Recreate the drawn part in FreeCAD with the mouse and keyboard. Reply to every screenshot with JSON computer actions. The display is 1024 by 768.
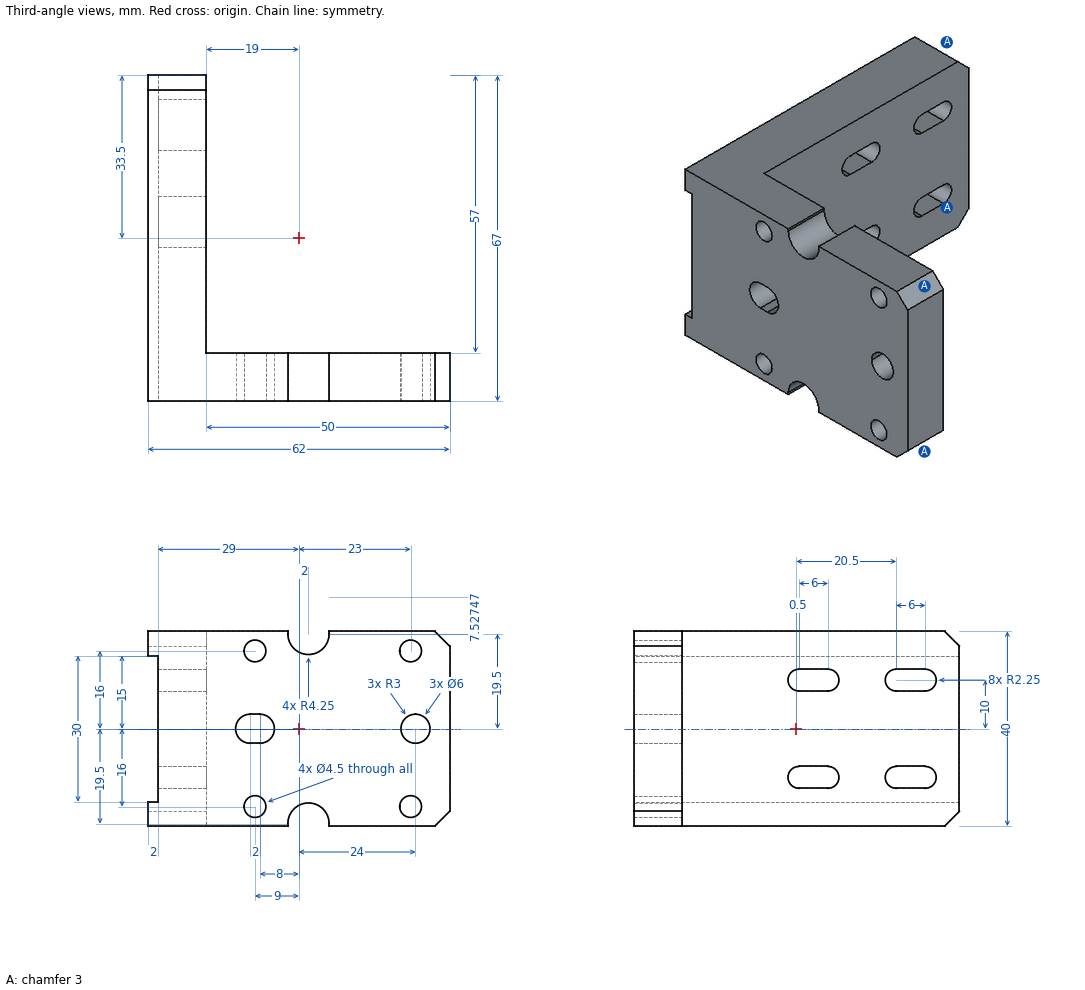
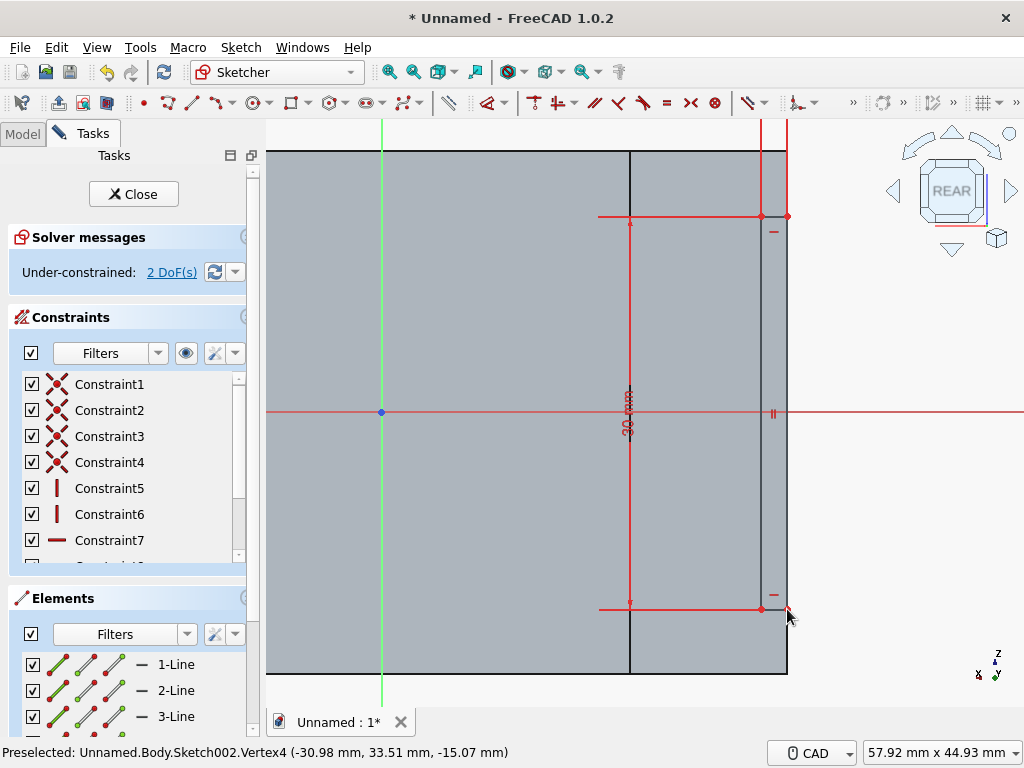
{"action": "left_click", "coordinate": [488, 104]}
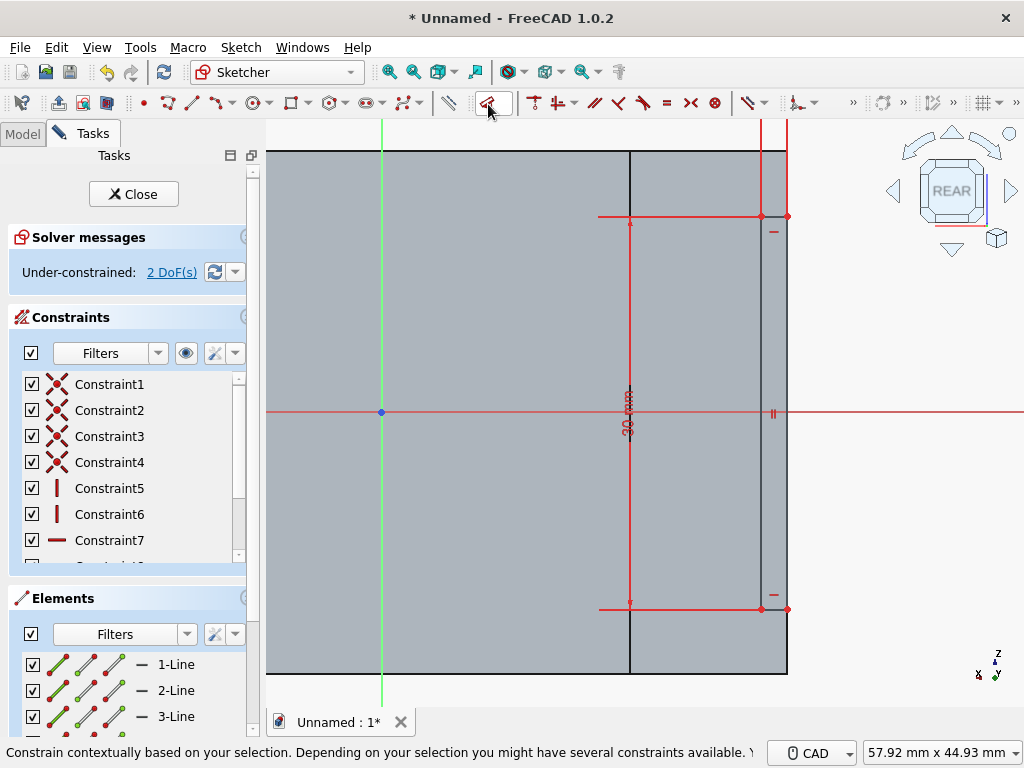
{"action": "left_click", "coordinate": [761, 217]}
{"action": "left_click", "coordinate": [571, 183]}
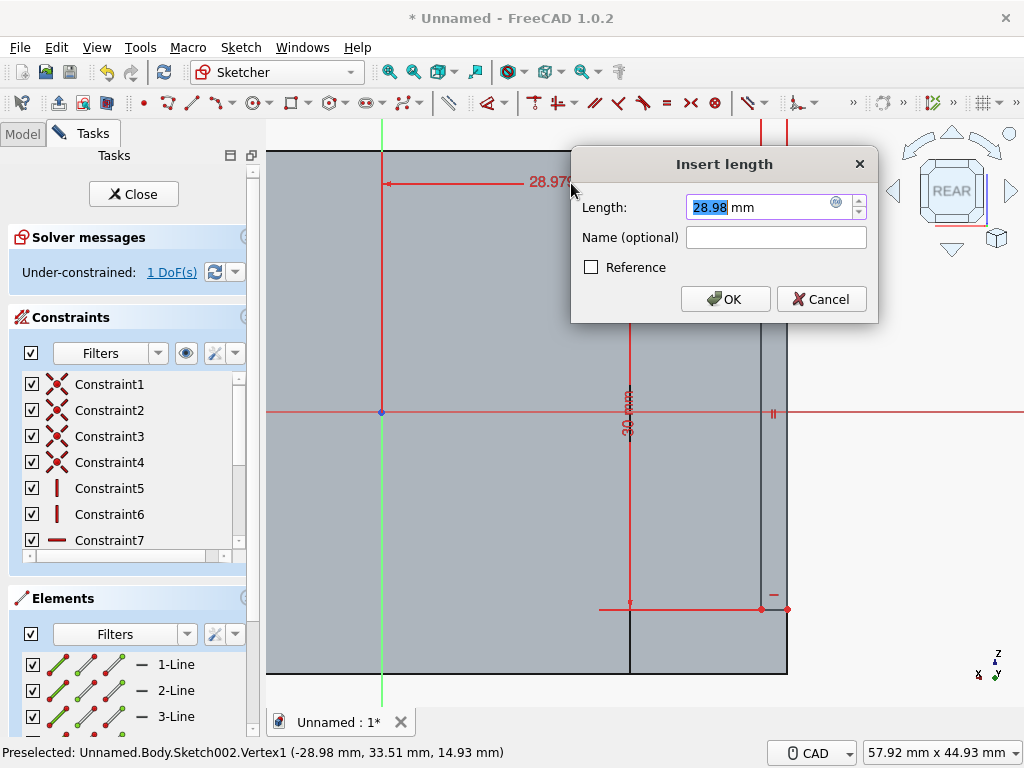
{"action": "type", "text": "29"}
{"action": "key", "text": "Return"}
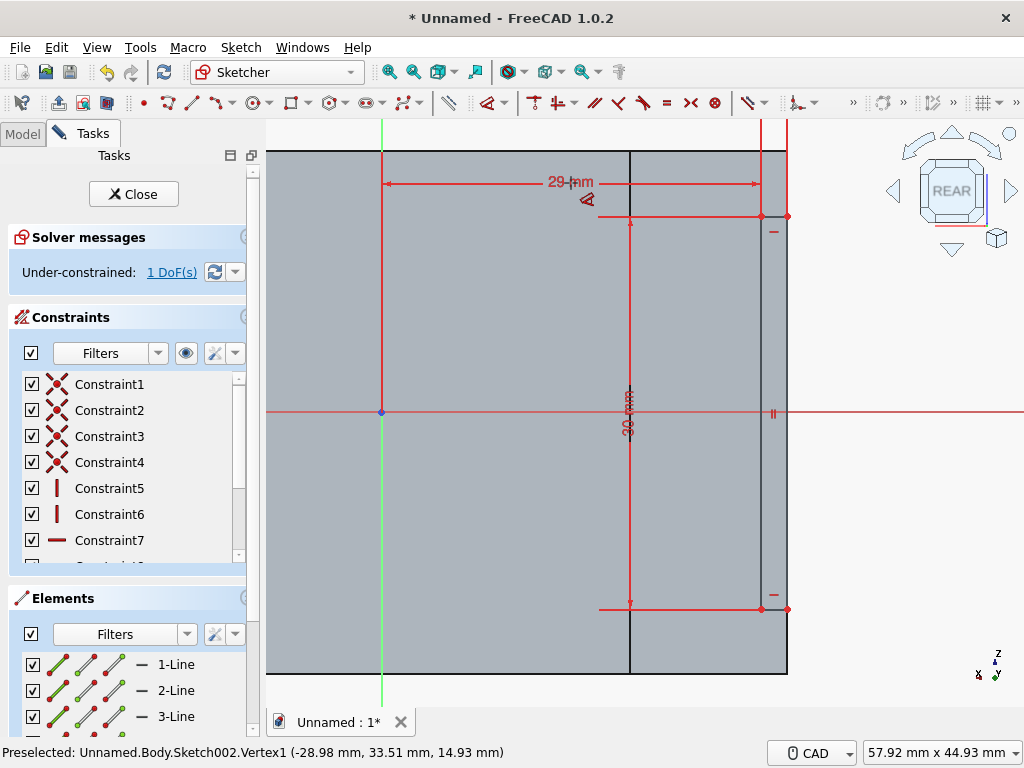
{"action": "left_click", "coordinate": [761, 217]}
{"action": "left_click", "coordinate": [348, 315]}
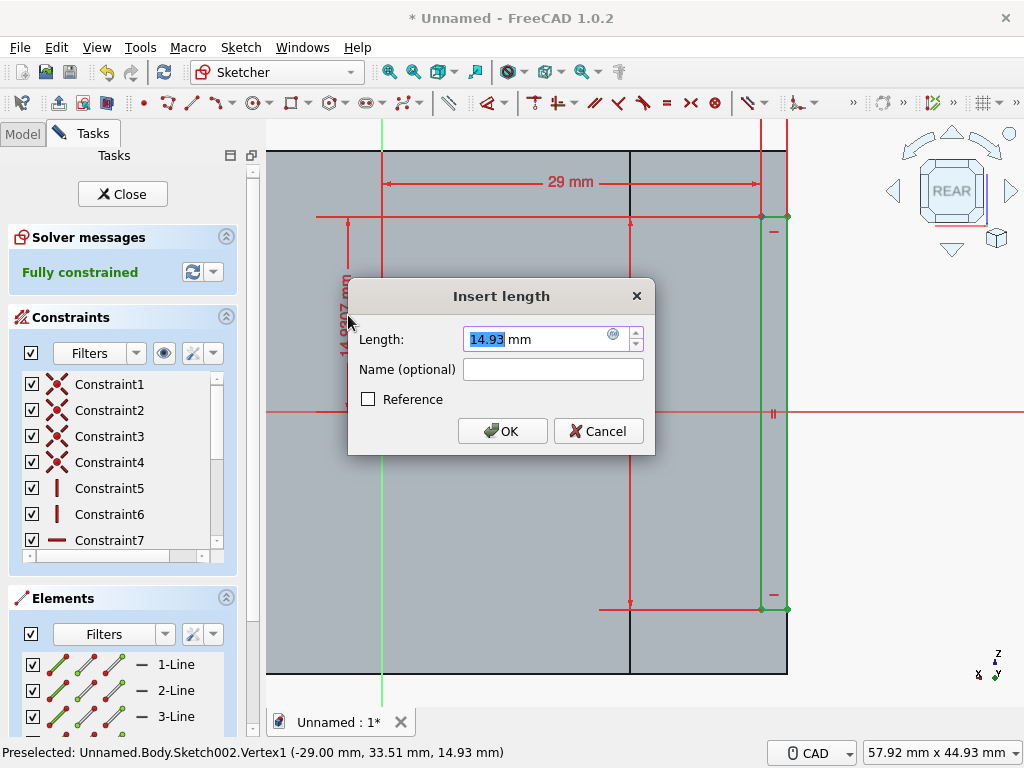
{"action": "type", "text": "15"}
{"action": "key", "text": "Return"}
{"action": "key", "text": "Escape"}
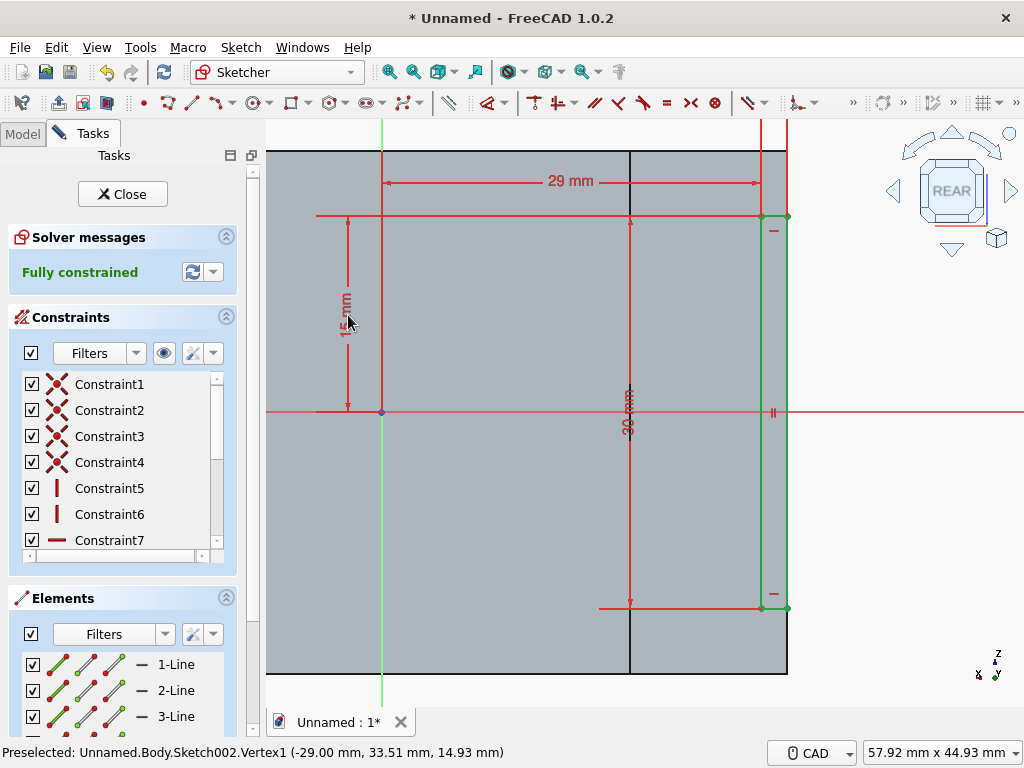
{"action": "left_click", "coordinate": [123, 194]}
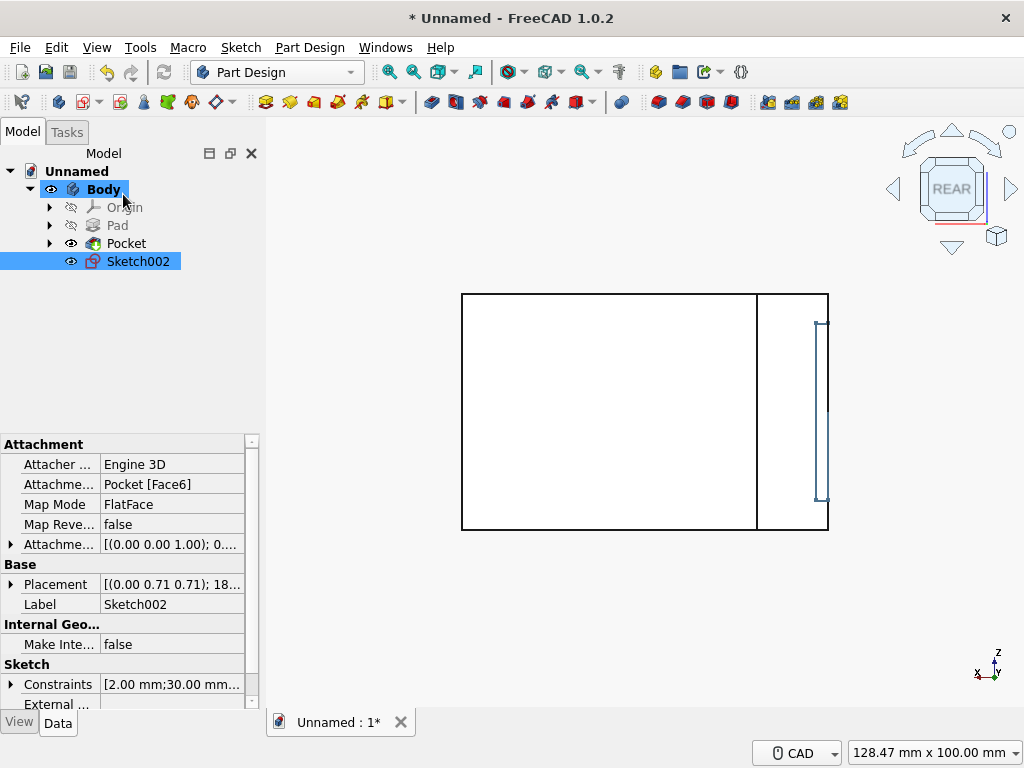
{"action": "left_click", "coordinate": [432, 102]}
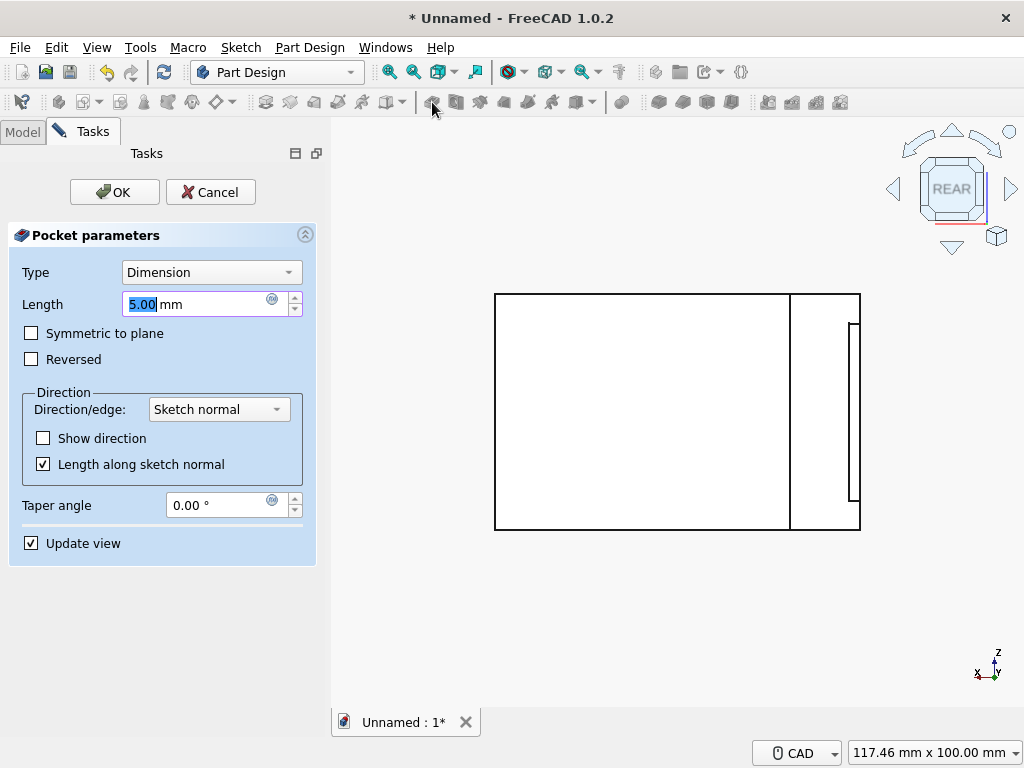
{"action": "left_click", "coordinate": [212, 272]}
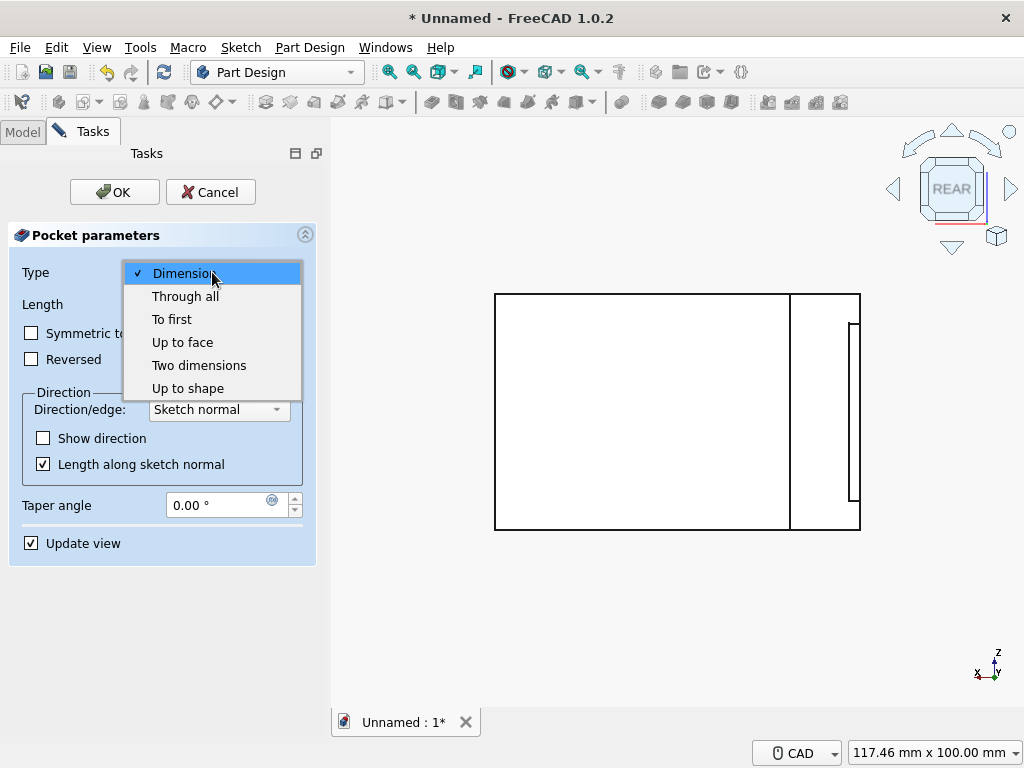
{"action": "left_click", "coordinate": [212, 296]}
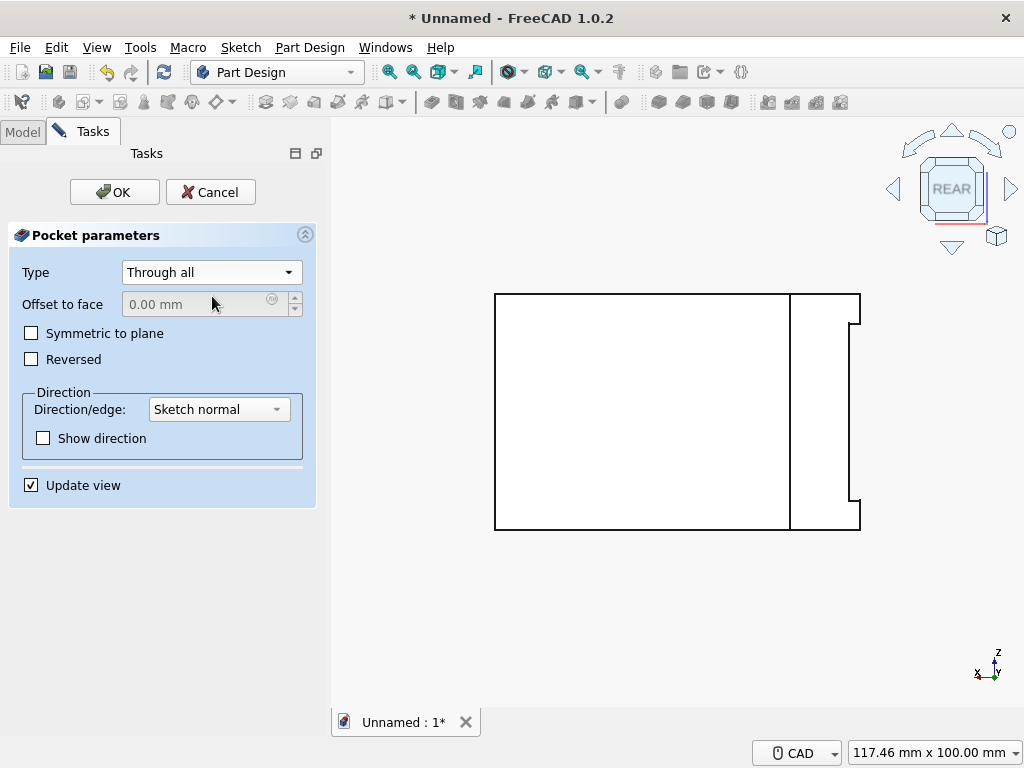
{"action": "left_click", "coordinate": [115, 192]}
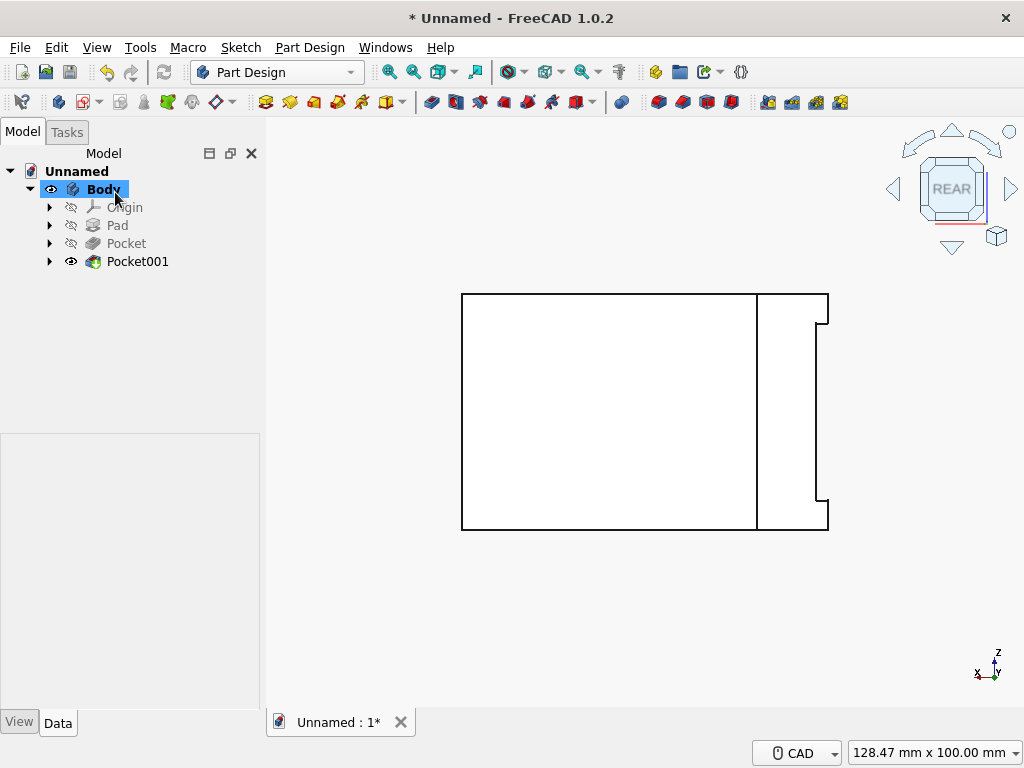
{"action": "key", "text": "0"}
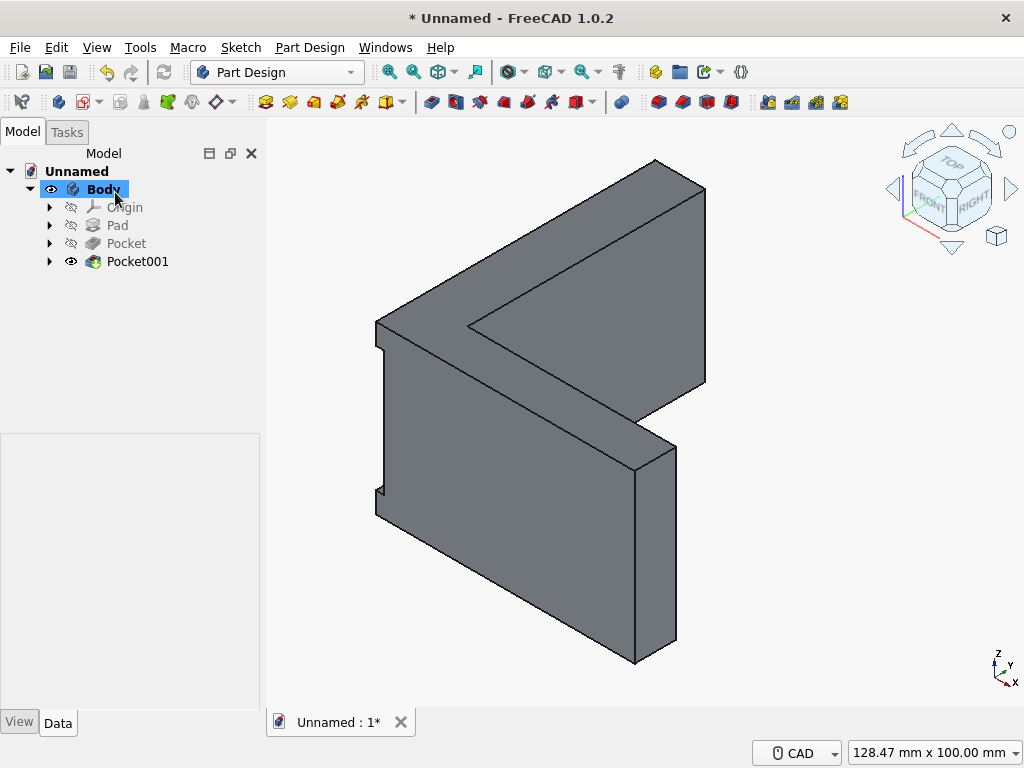
{"action": "left_click", "coordinate": [621, 334]}